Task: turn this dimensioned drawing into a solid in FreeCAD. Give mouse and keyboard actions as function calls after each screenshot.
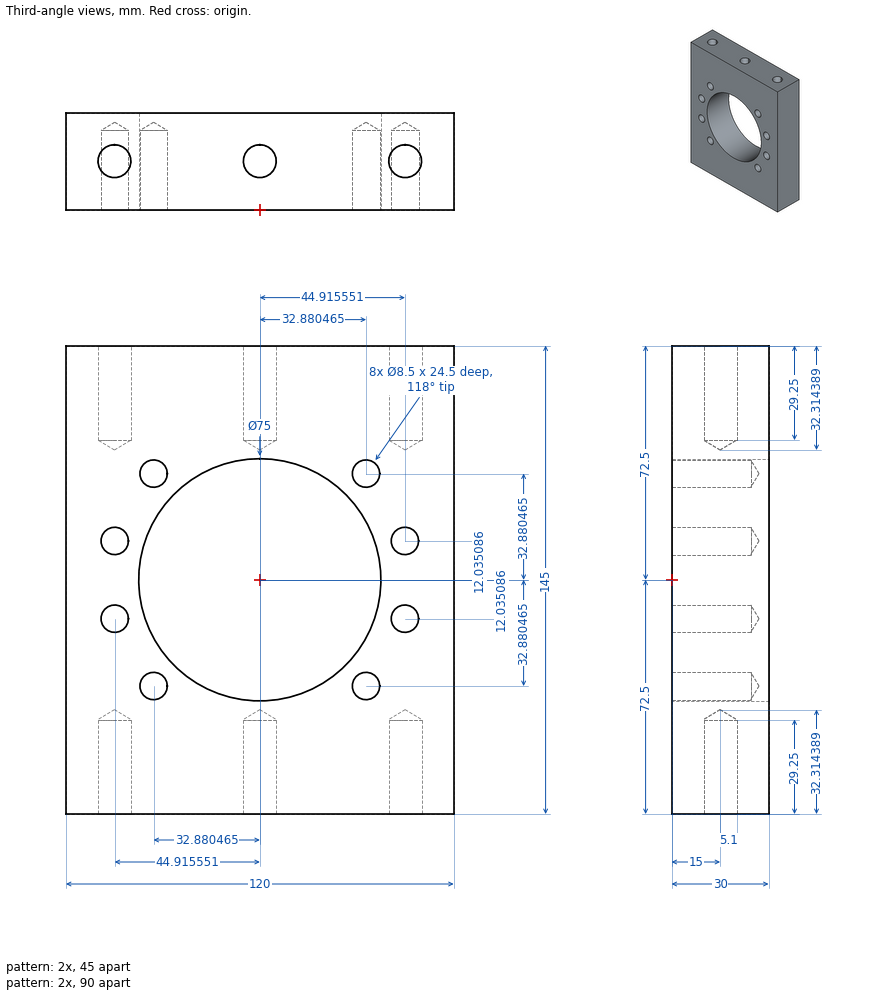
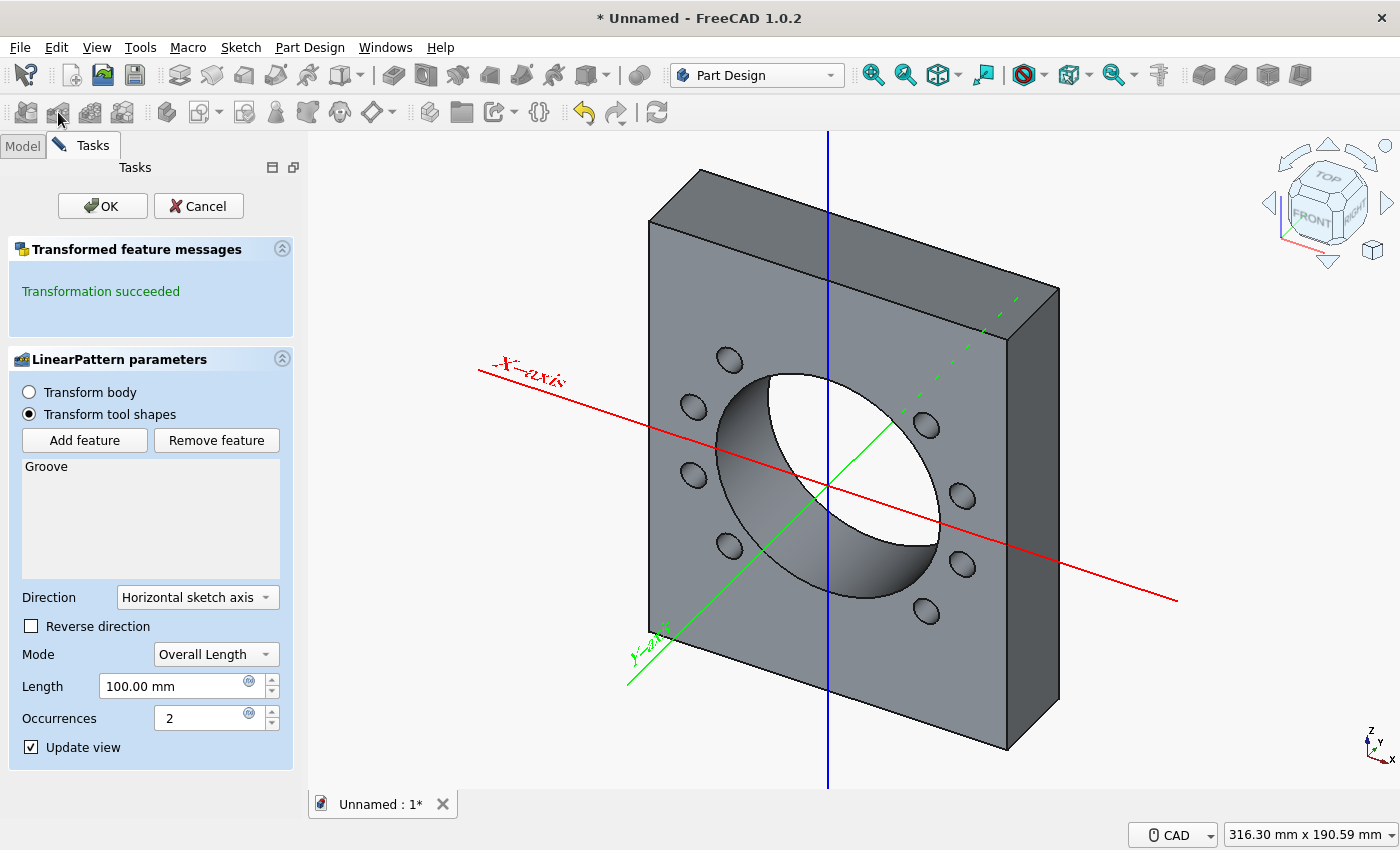
click(198, 598)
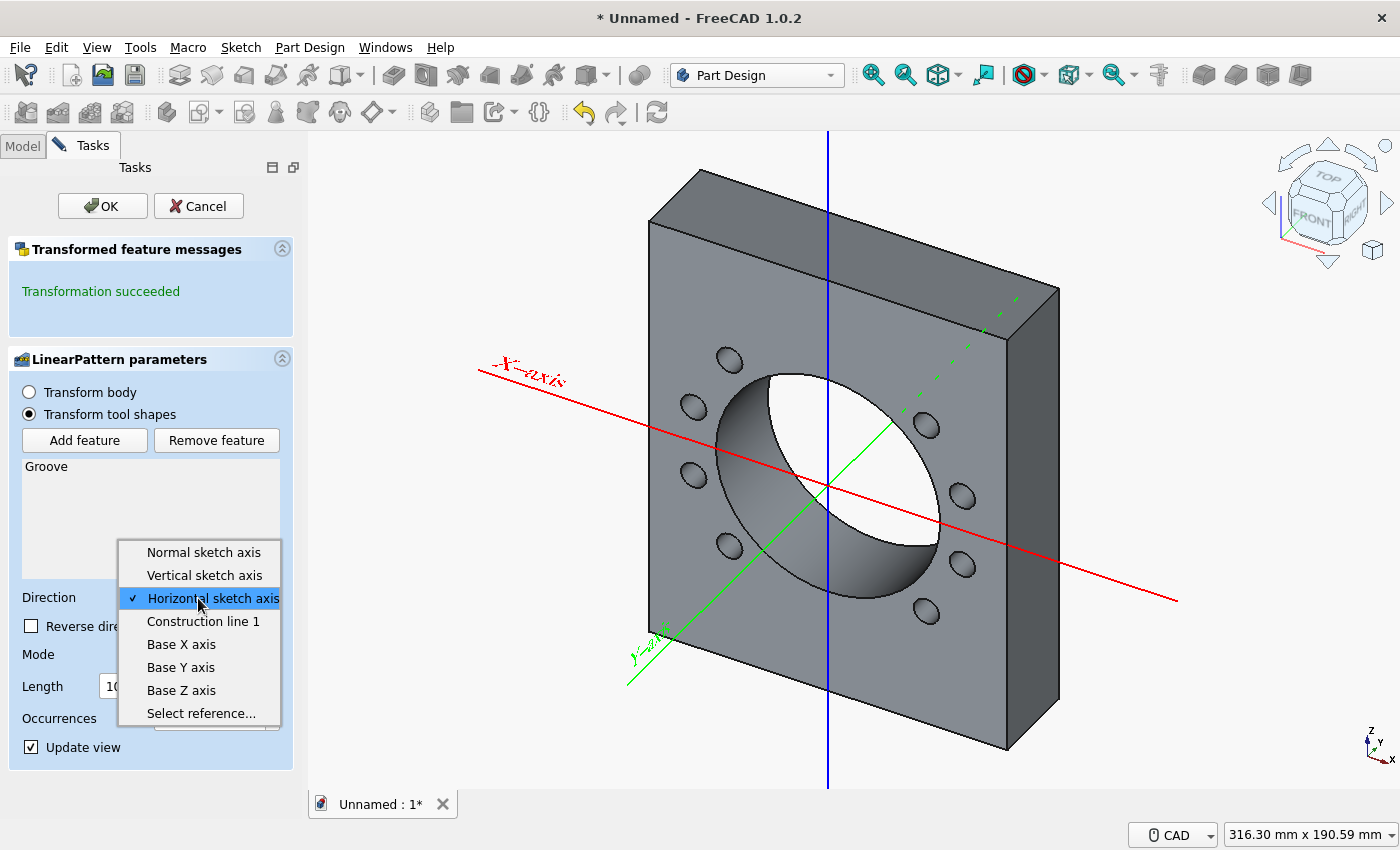
click(198, 644)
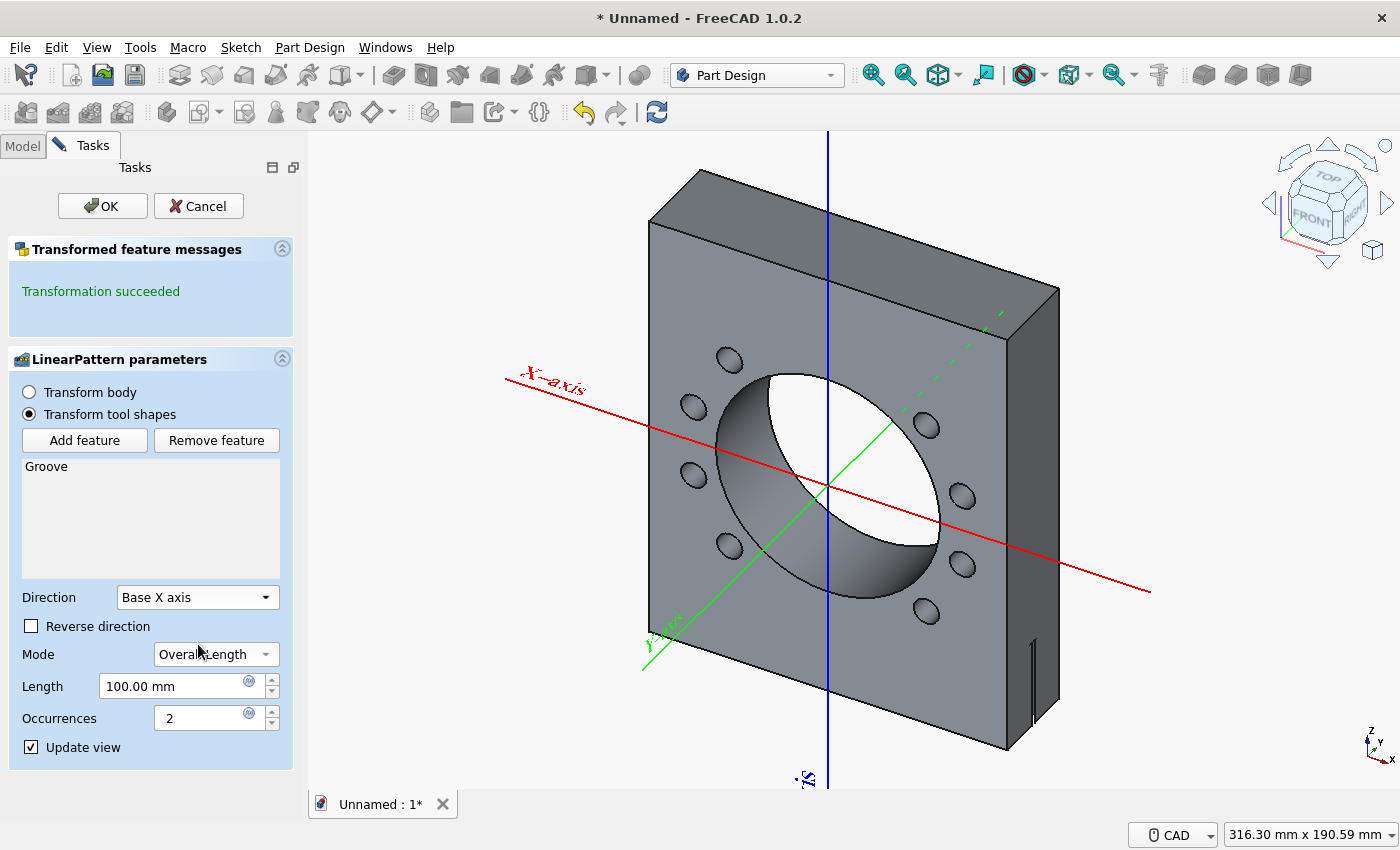
click(217, 654)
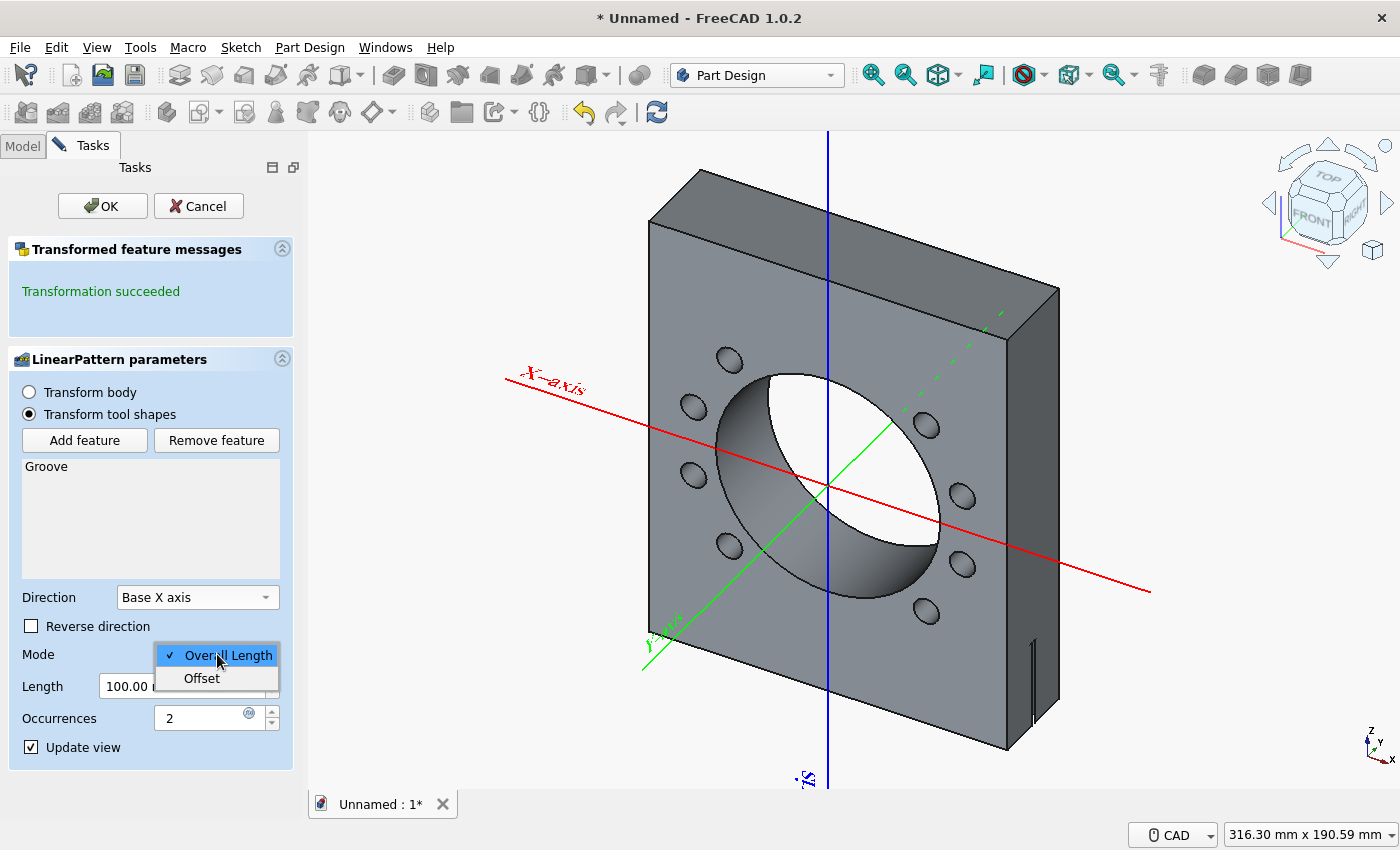
click(216, 678)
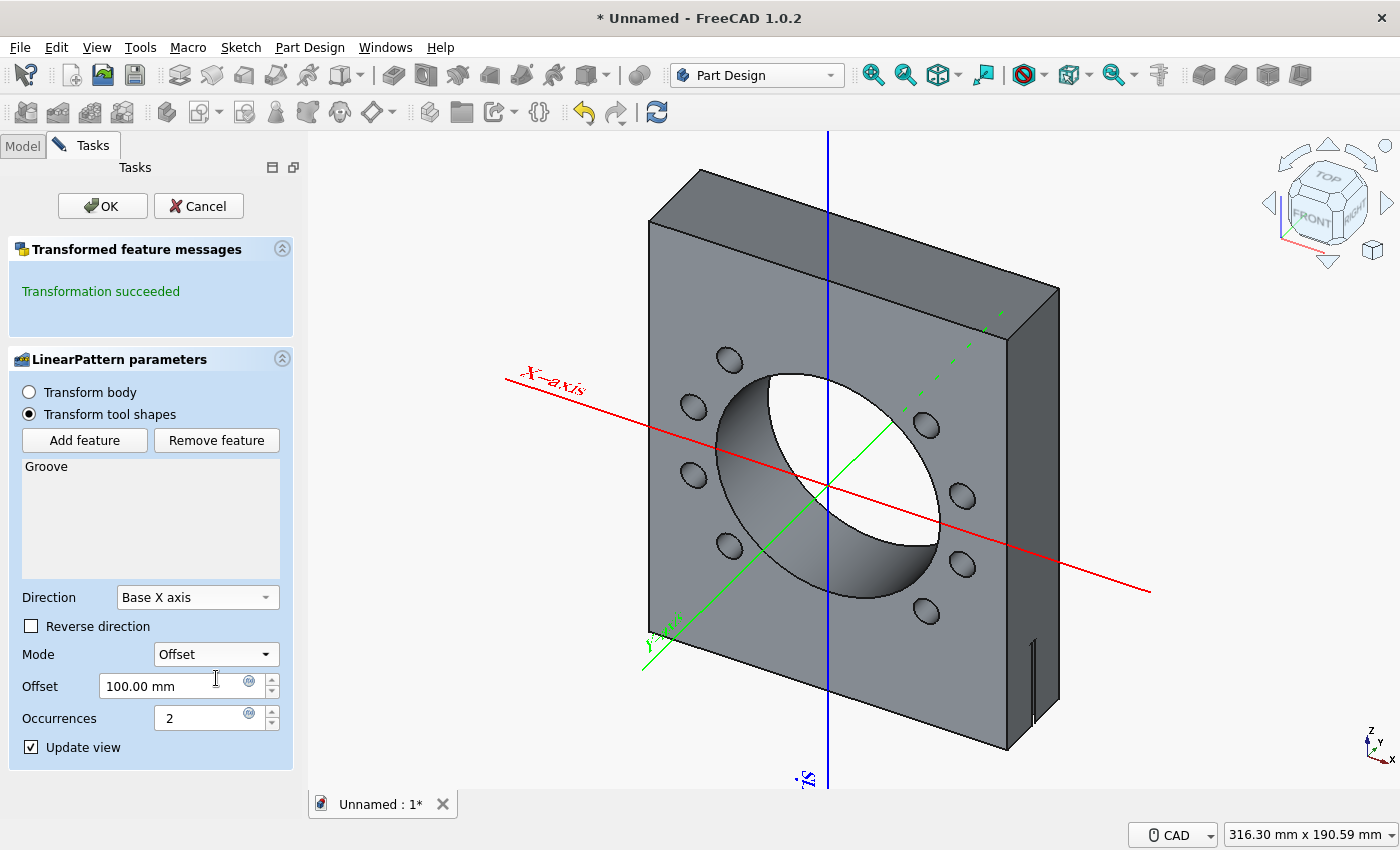
triple_click(182, 686)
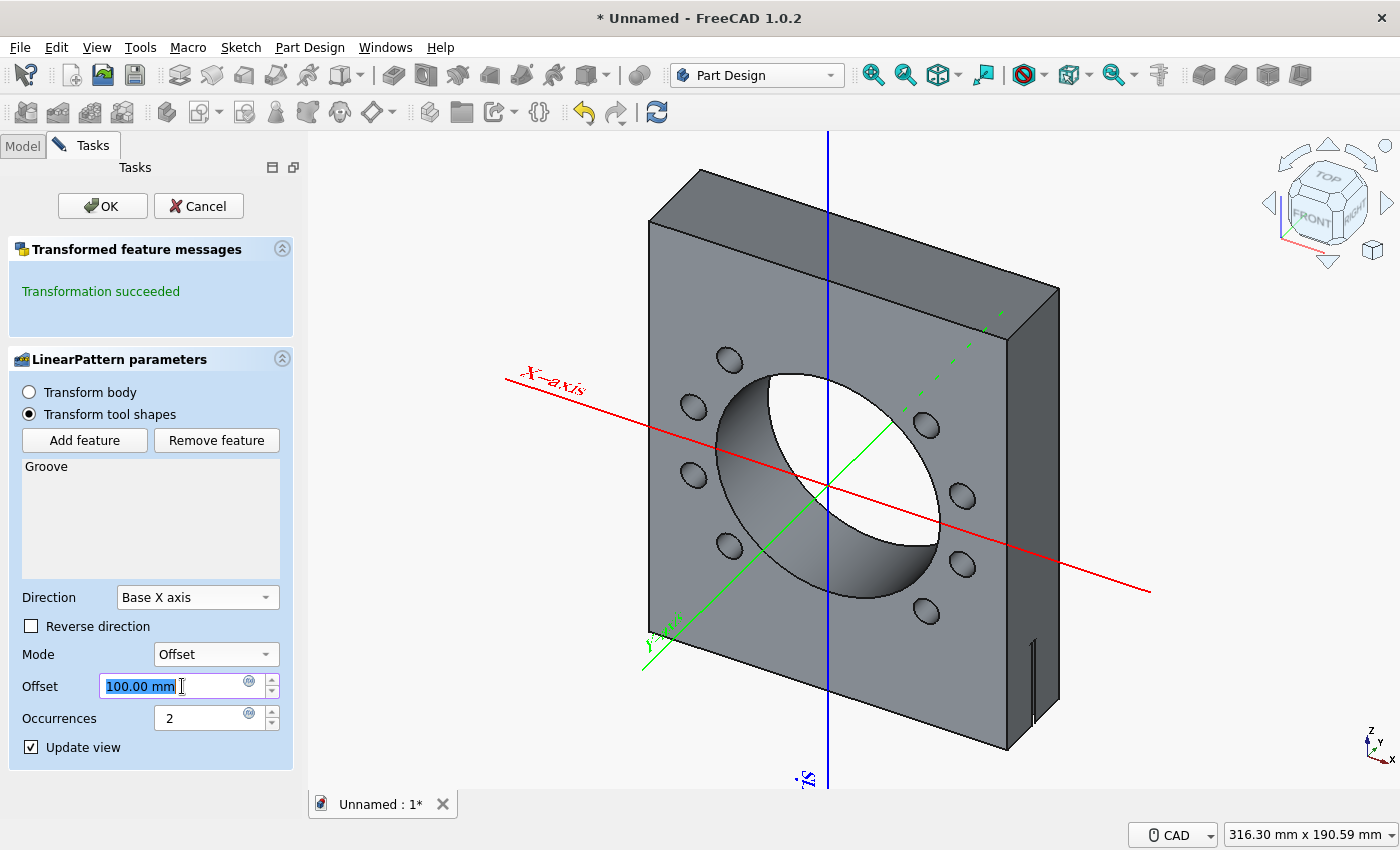
text(90)
key(Tab)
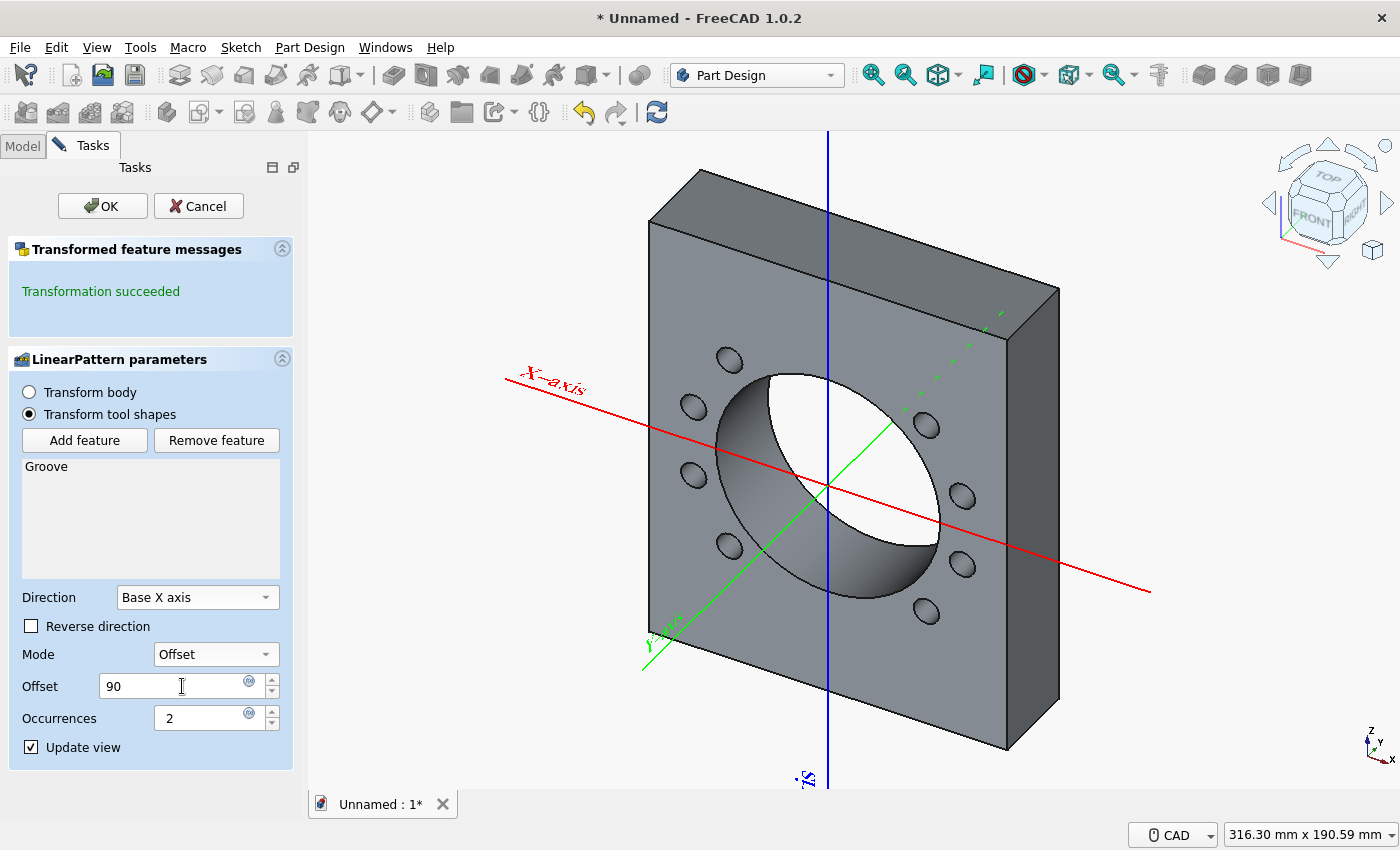
triple_click(209, 718)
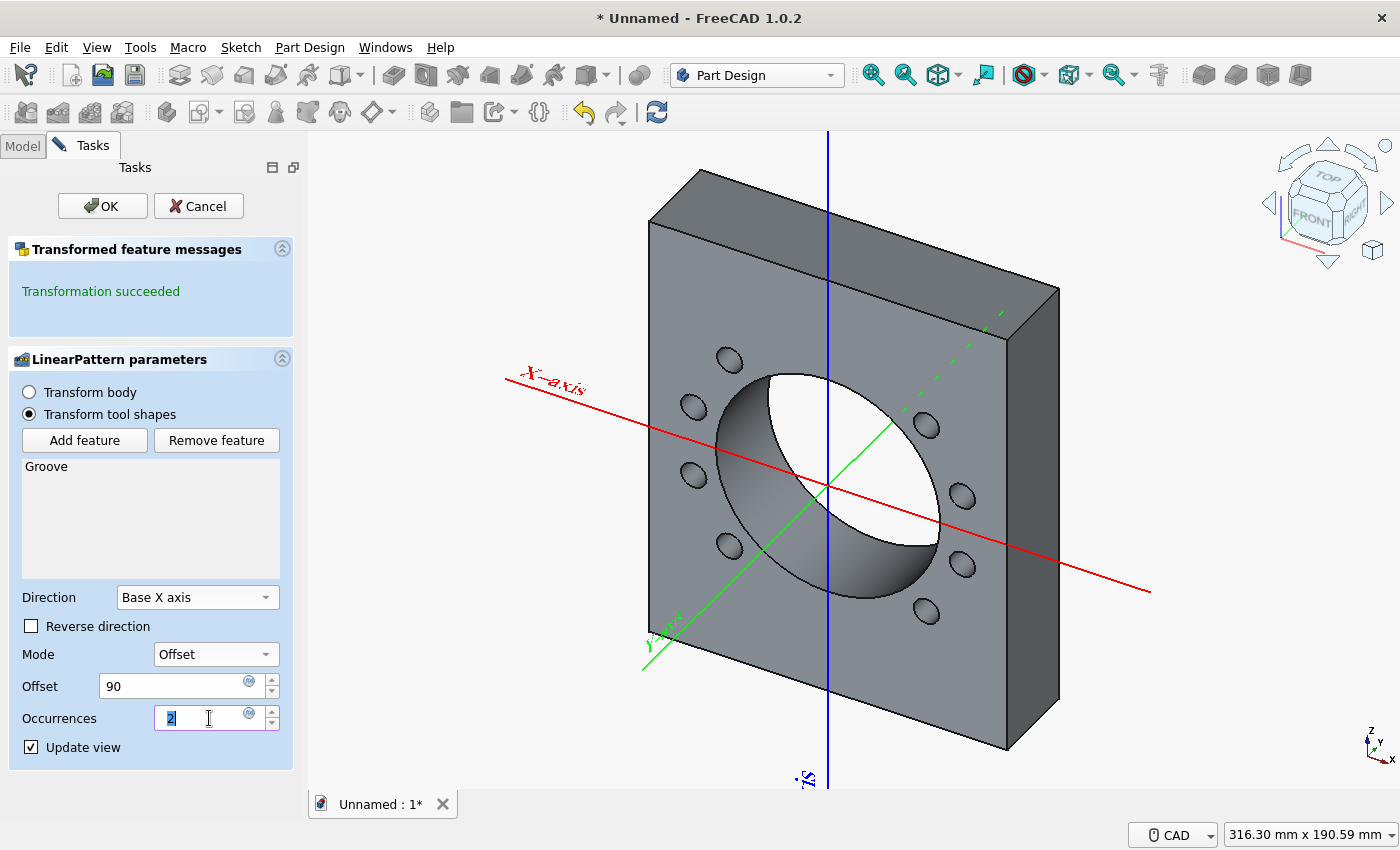
text(2)
key(Tab)